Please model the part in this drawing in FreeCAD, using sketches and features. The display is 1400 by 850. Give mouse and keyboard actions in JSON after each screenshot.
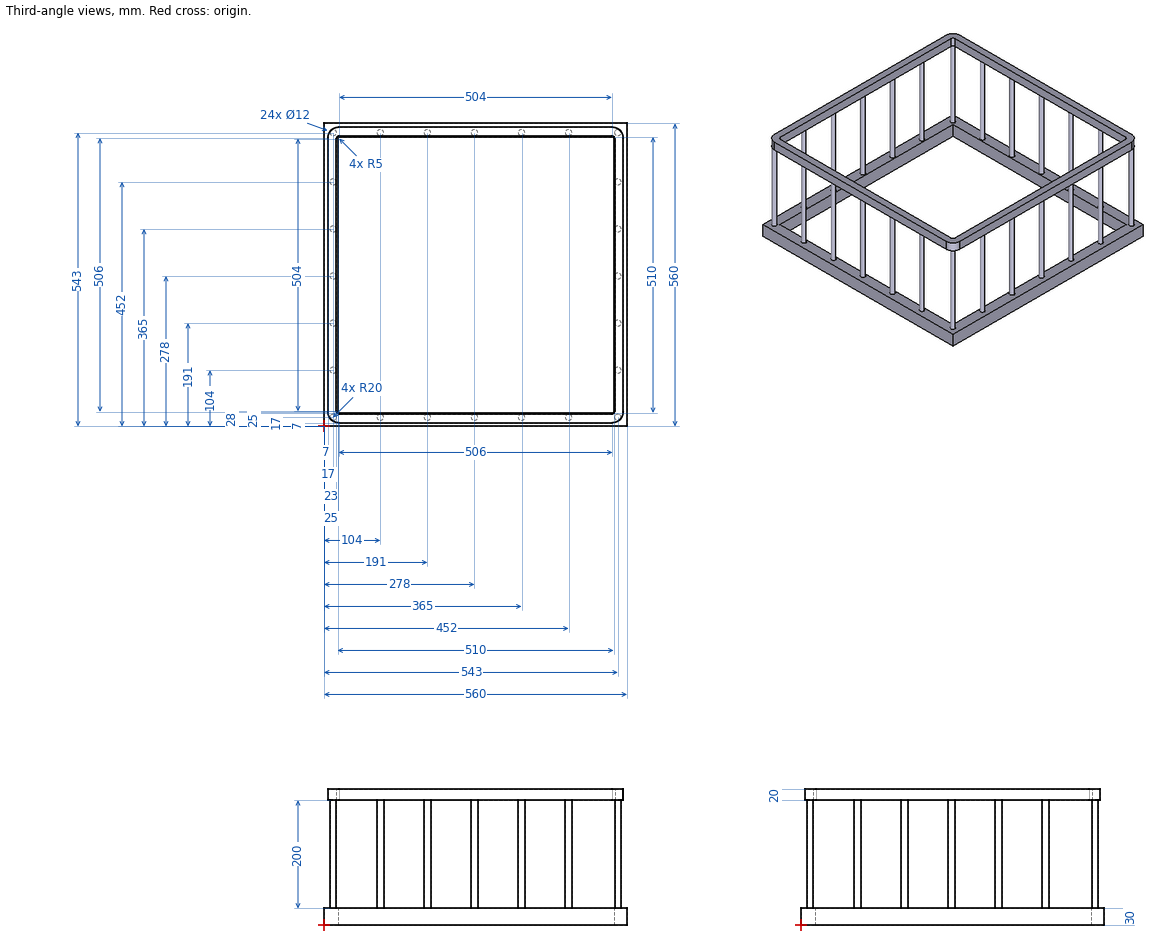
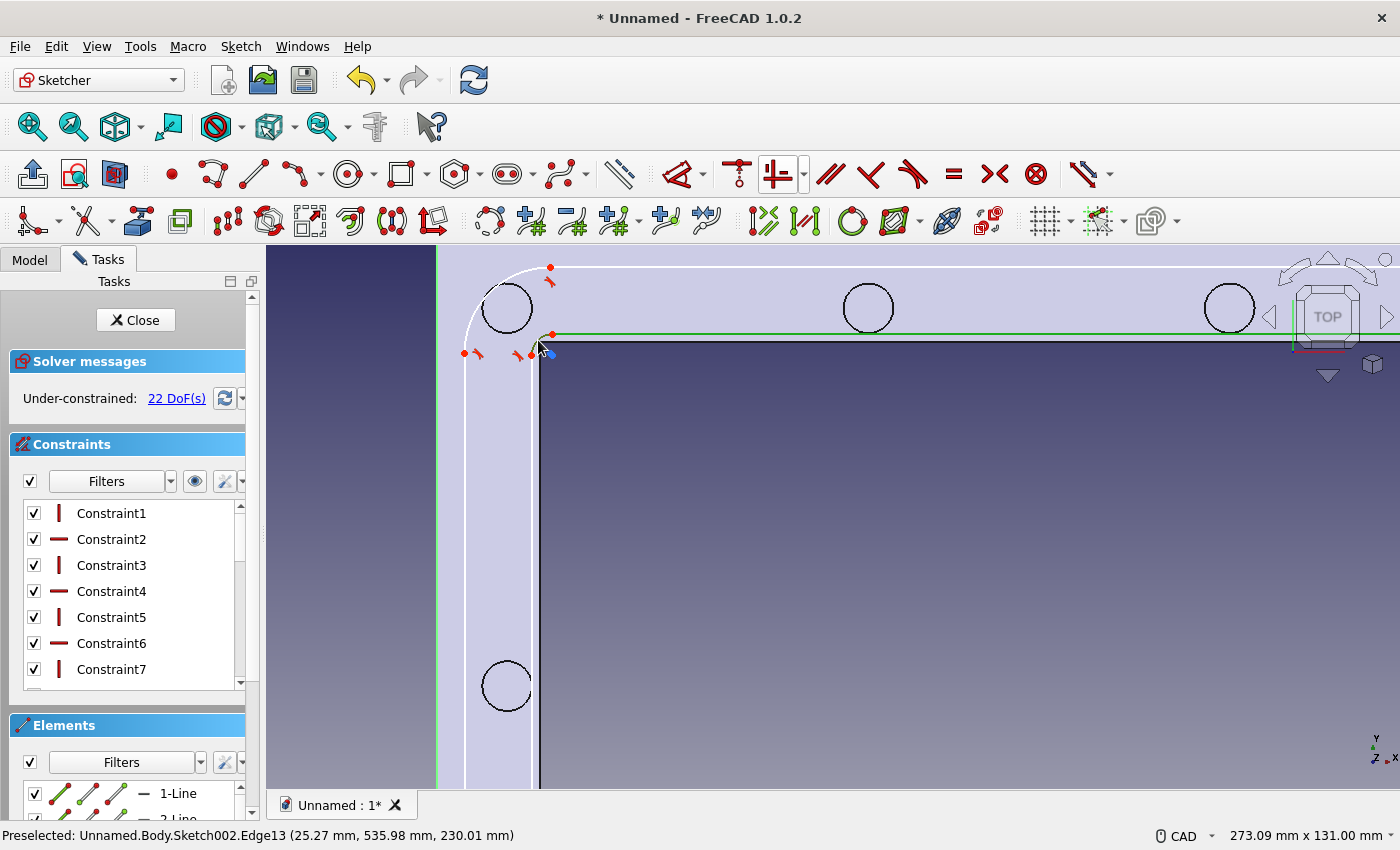
{"action": "left_click", "coordinate": [913, 174]}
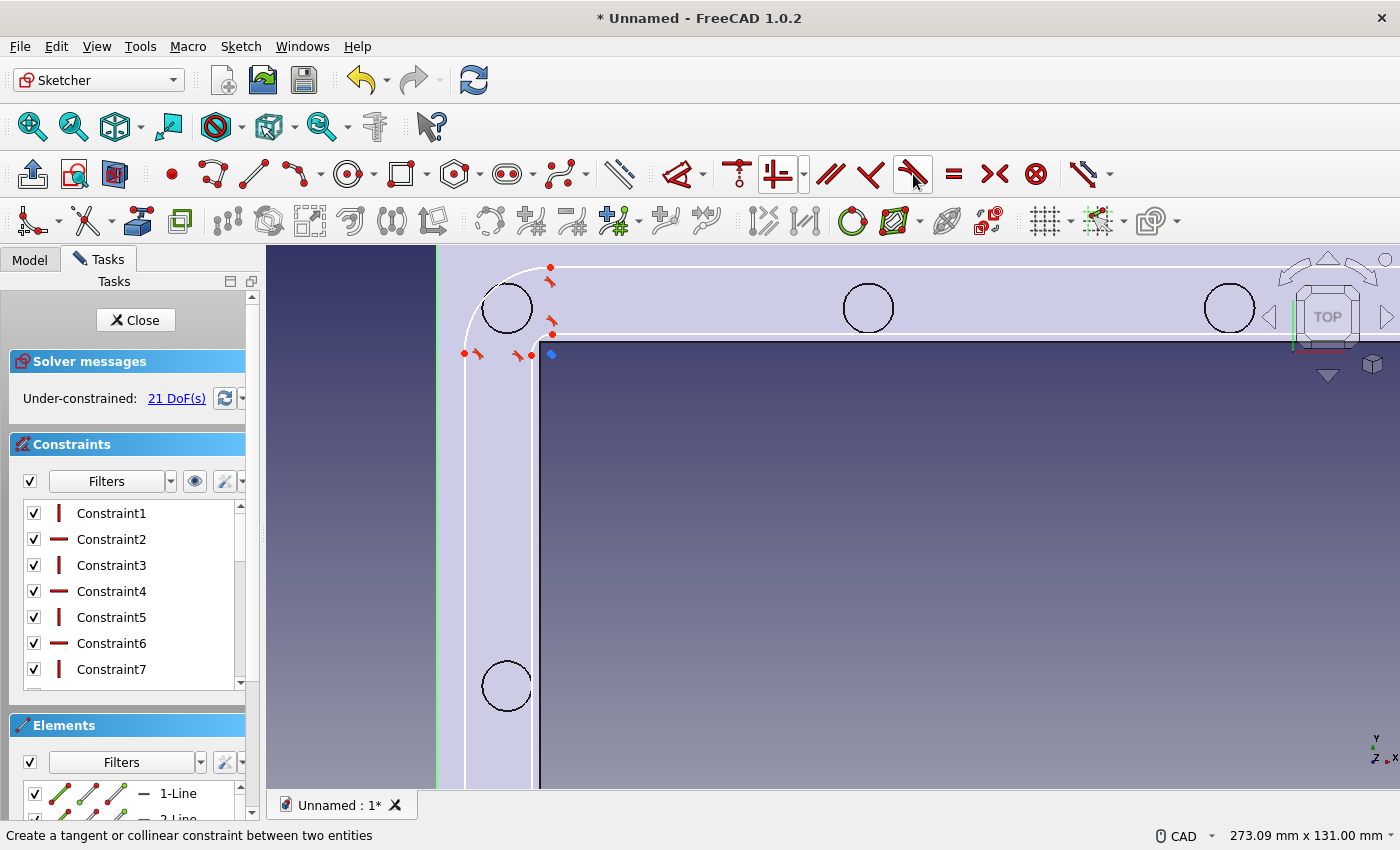
{"action": "scroll", "coordinate": [602, 339], "scroll_direction": "down", "scroll_amount": 9}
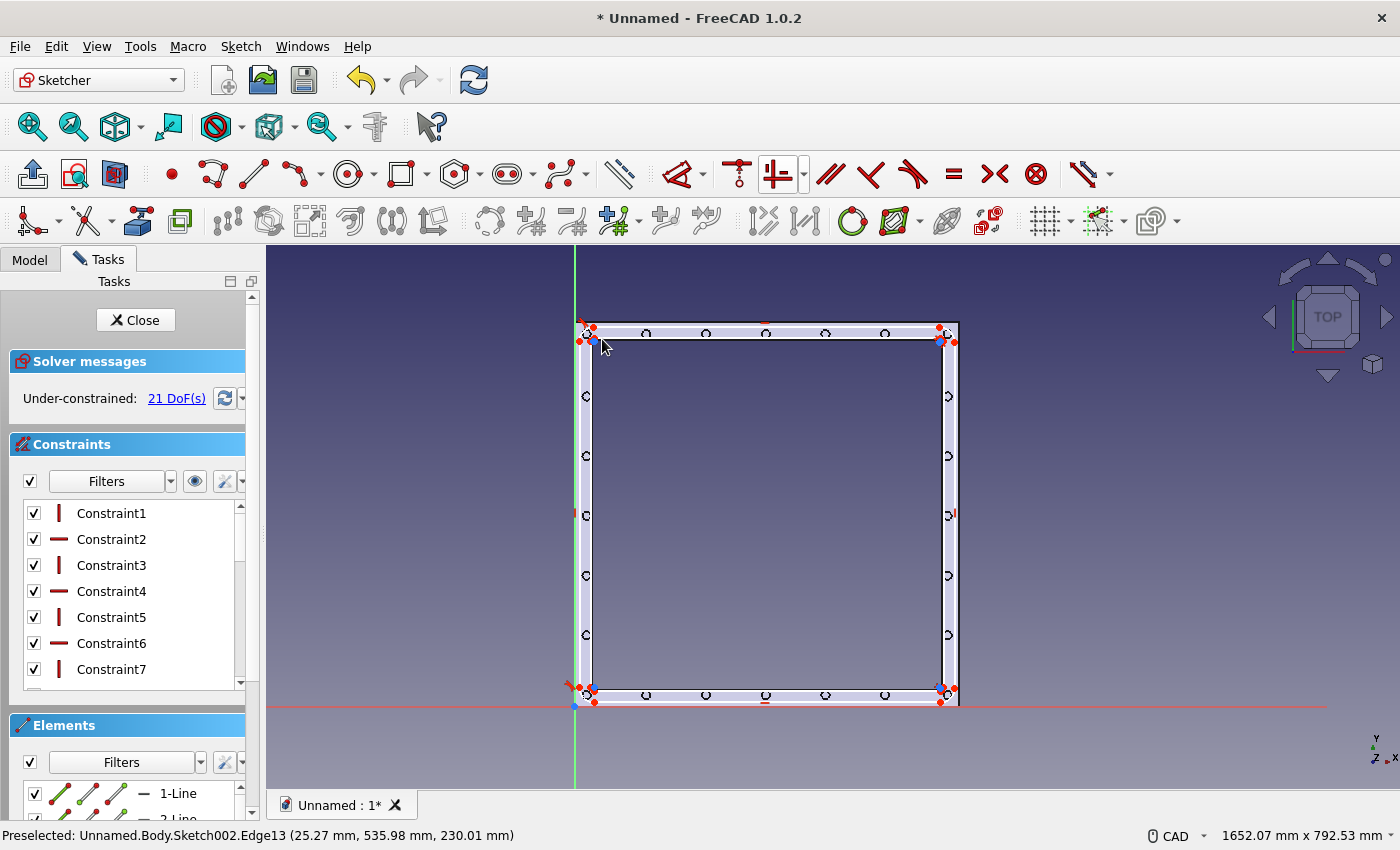
{"action": "scroll", "coordinate": [698, 338], "scroll_direction": "up", "scroll_amount": 2}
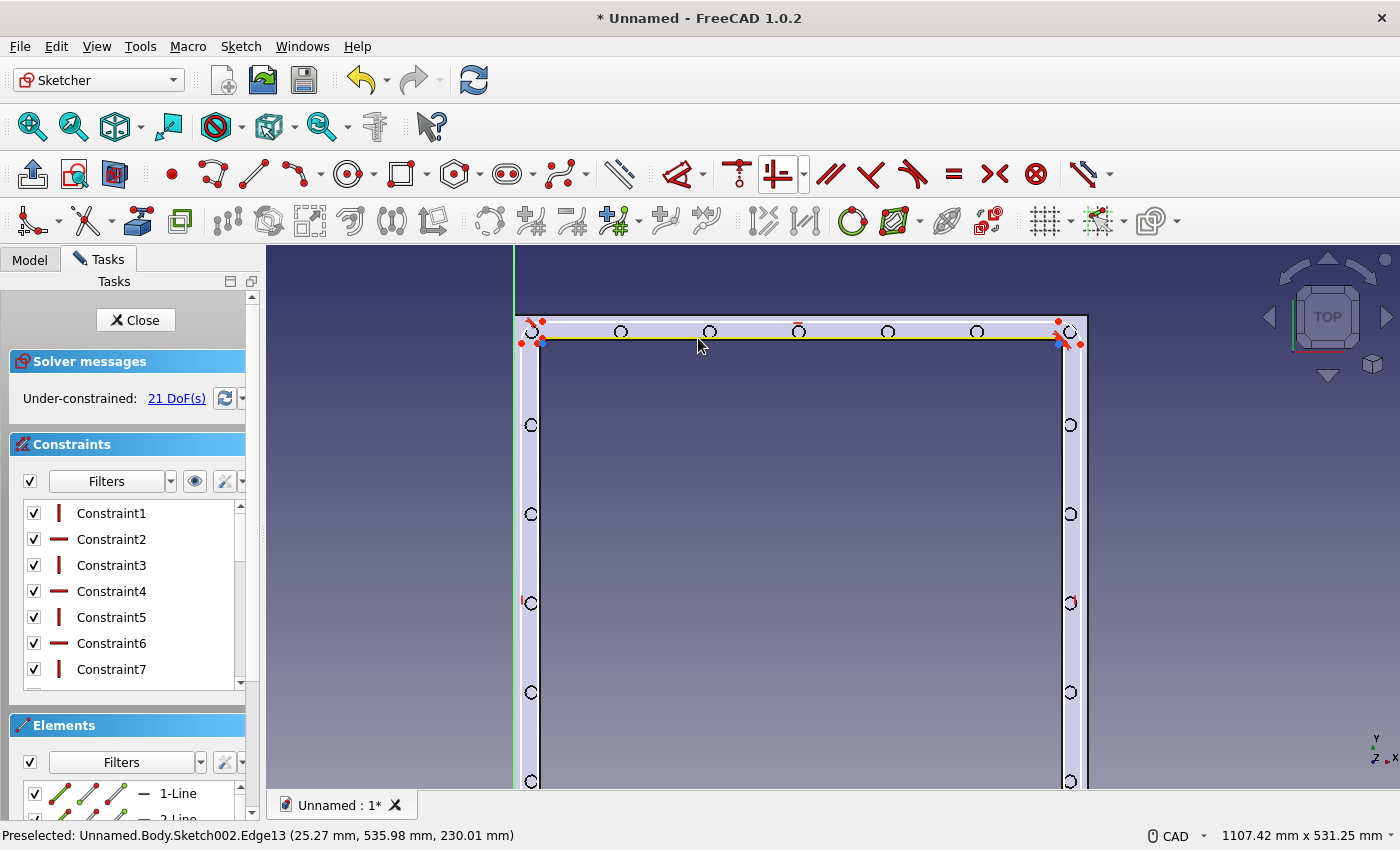
{"action": "left_click", "coordinate": [698, 338]}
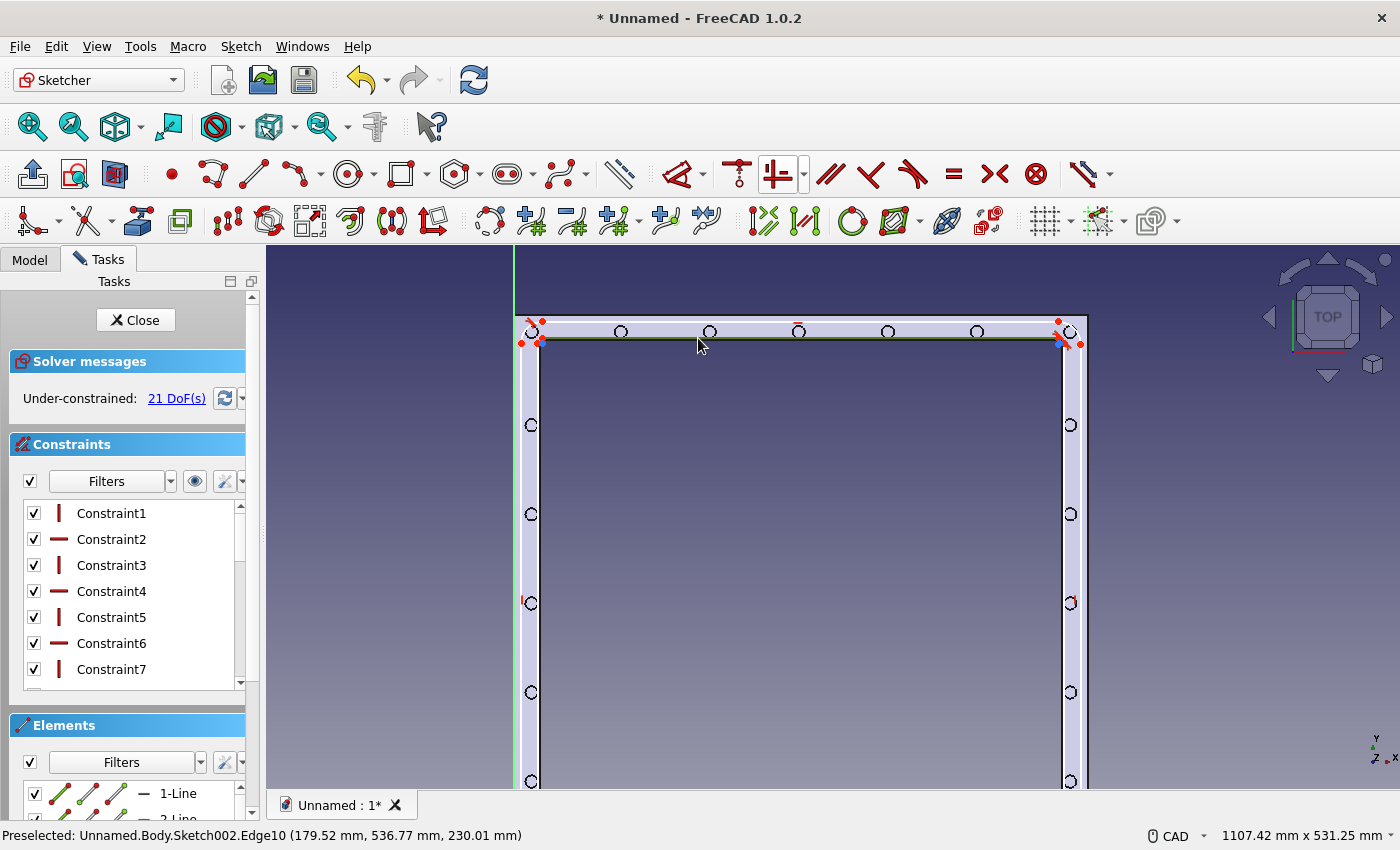
{"action": "scroll", "coordinate": [1063, 340], "scroll_direction": "up", "scroll_amount": 7}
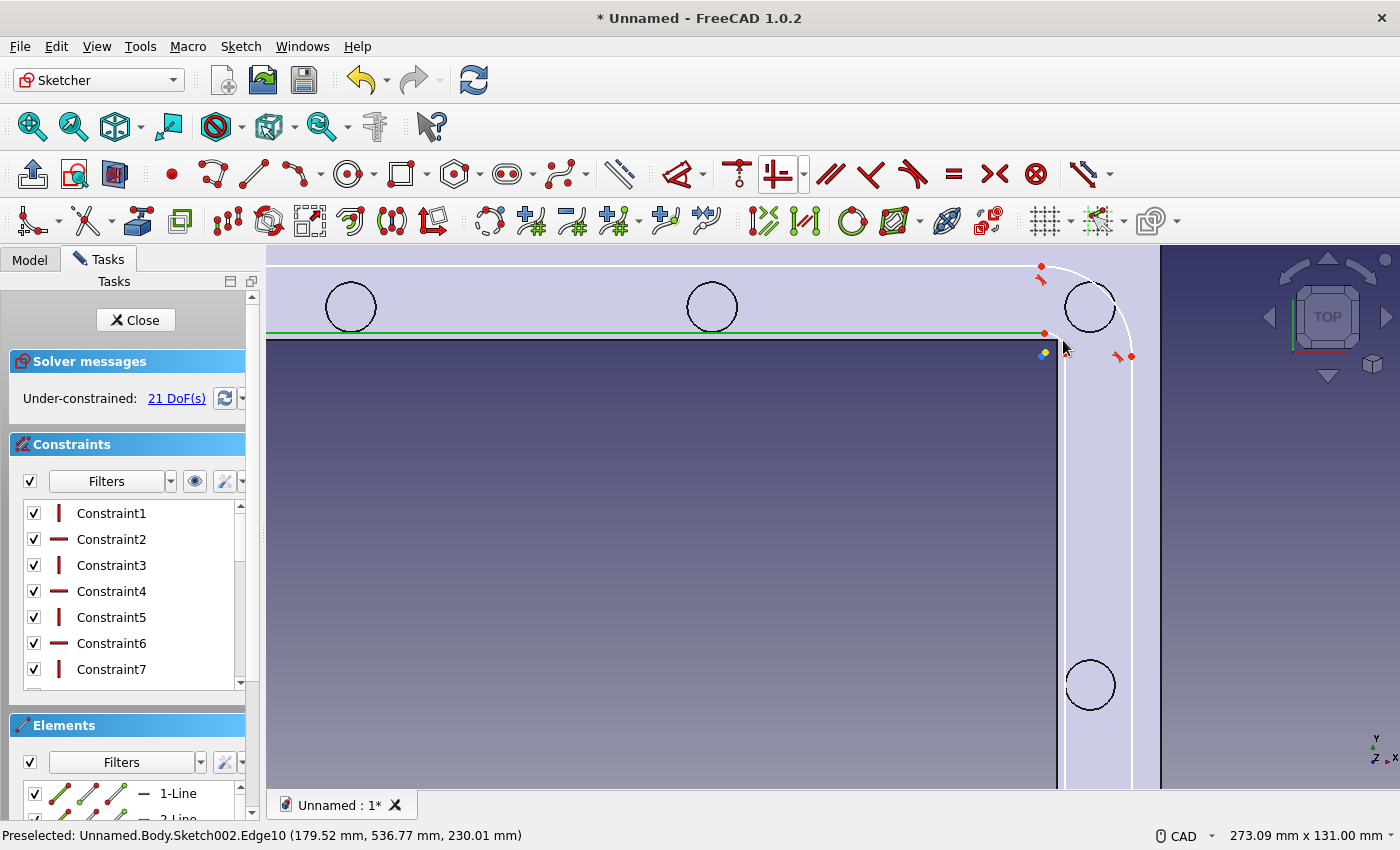
{"action": "left_click", "coordinate": [1060, 339]}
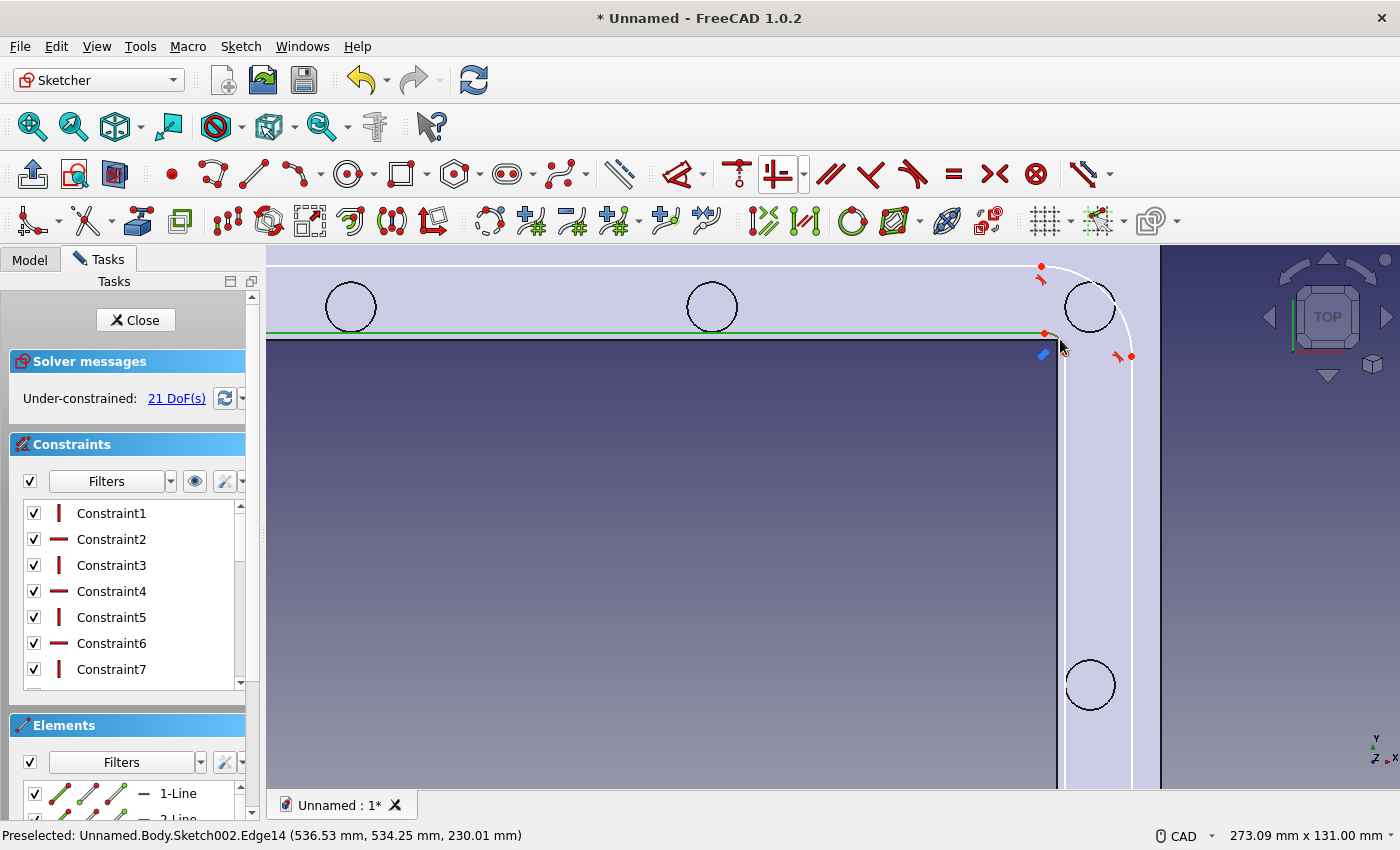
{"action": "left_click", "coordinate": [913, 174]}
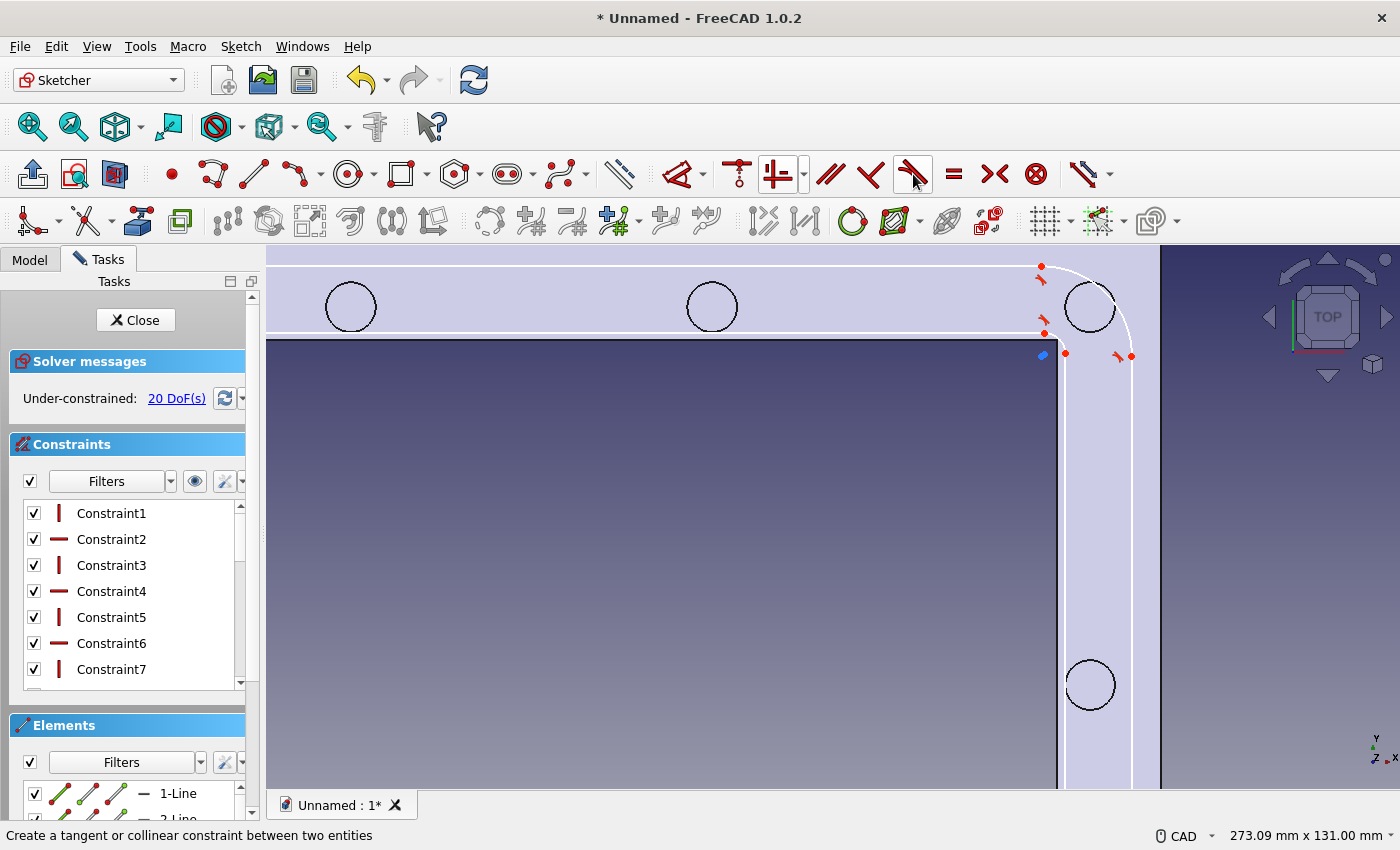
{"action": "scroll", "coordinate": [919, 339], "scroll_direction": "down", "scroll_amount": 9}